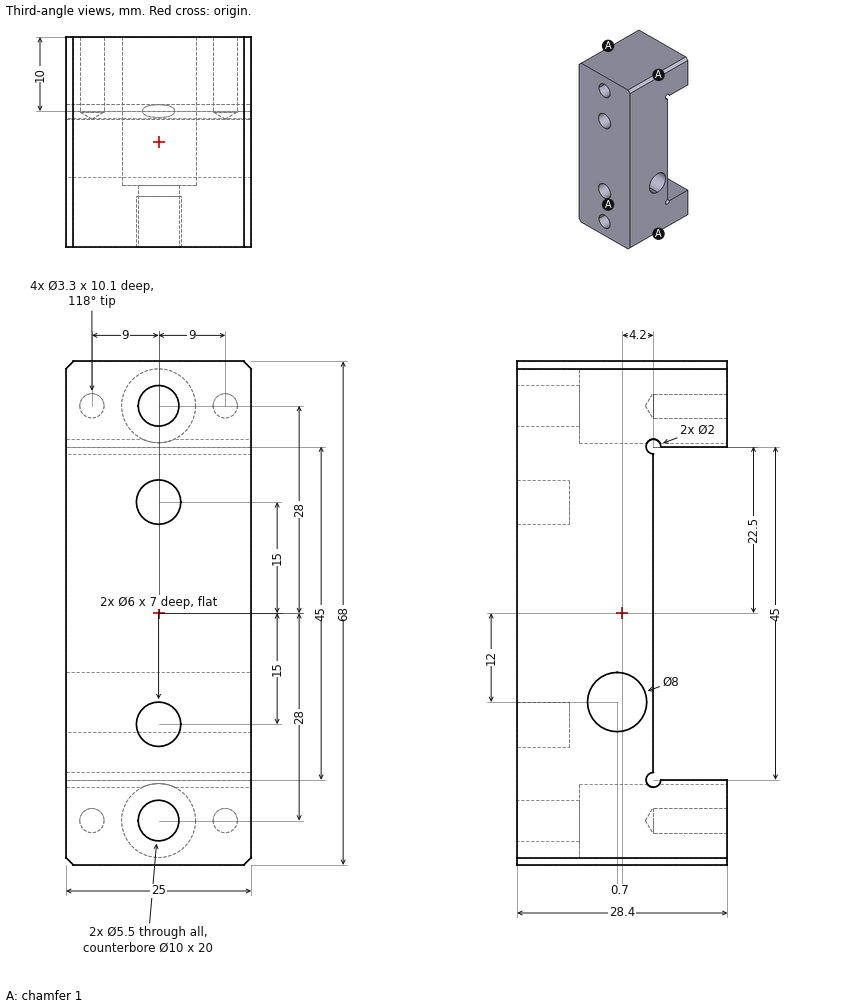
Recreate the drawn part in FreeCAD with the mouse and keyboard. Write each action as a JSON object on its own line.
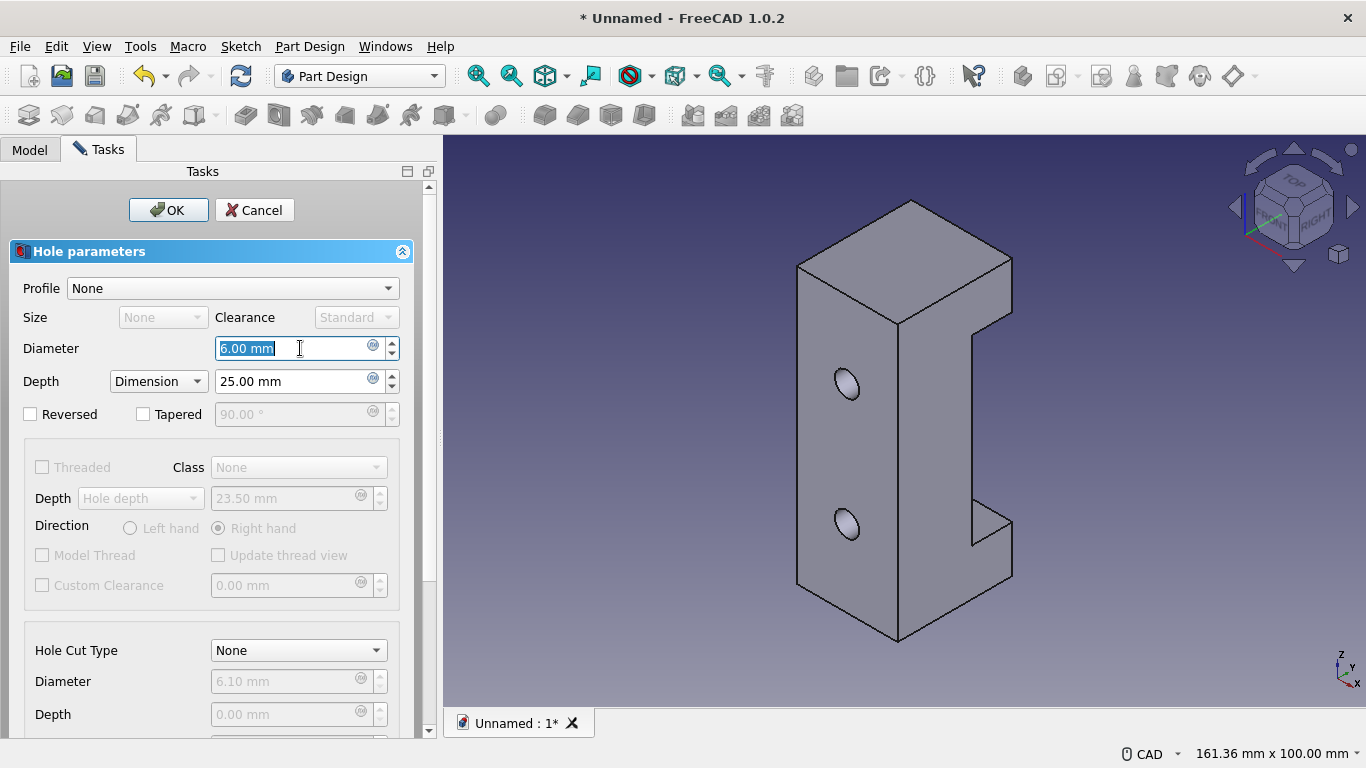
{"action": "type", "text": "6"}
{"action": "key", "text": "Tab"}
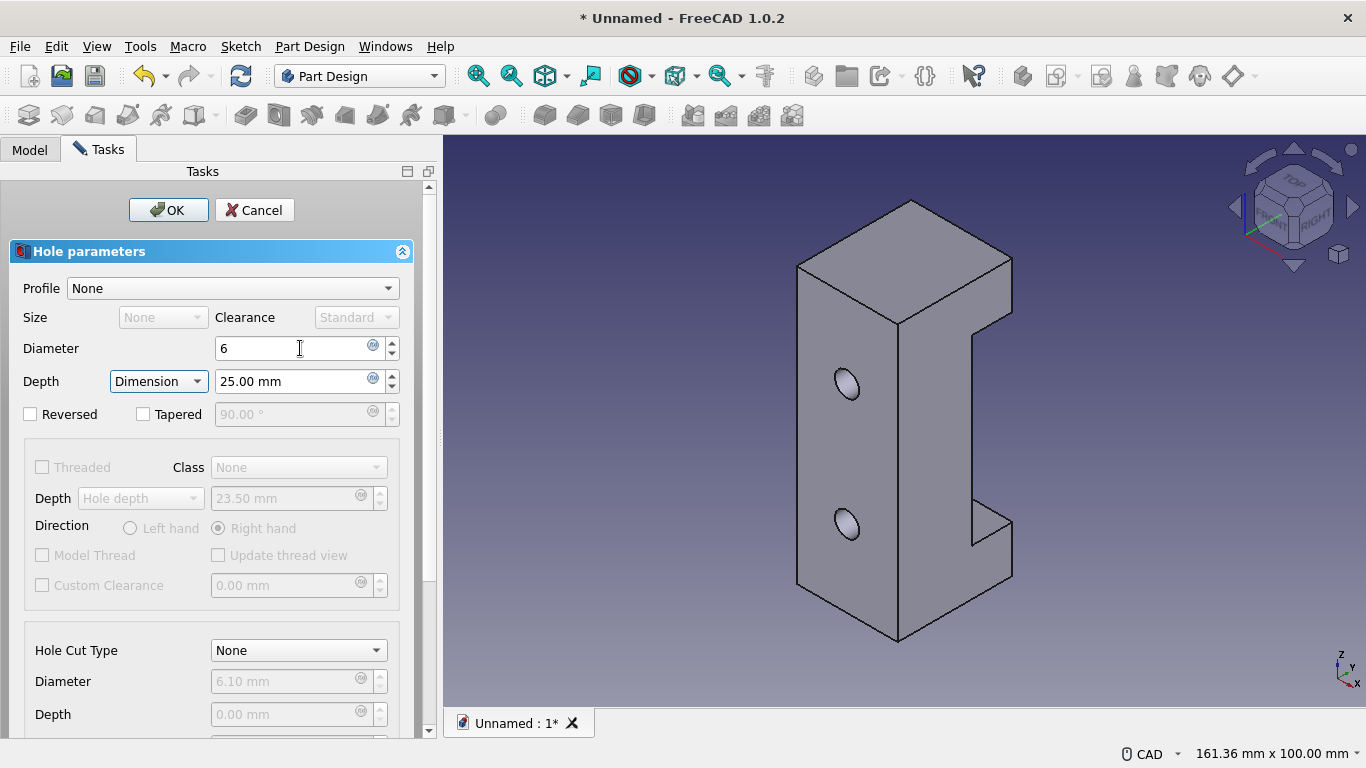
{"action": "triple_click", "coordinate": [300, 382]}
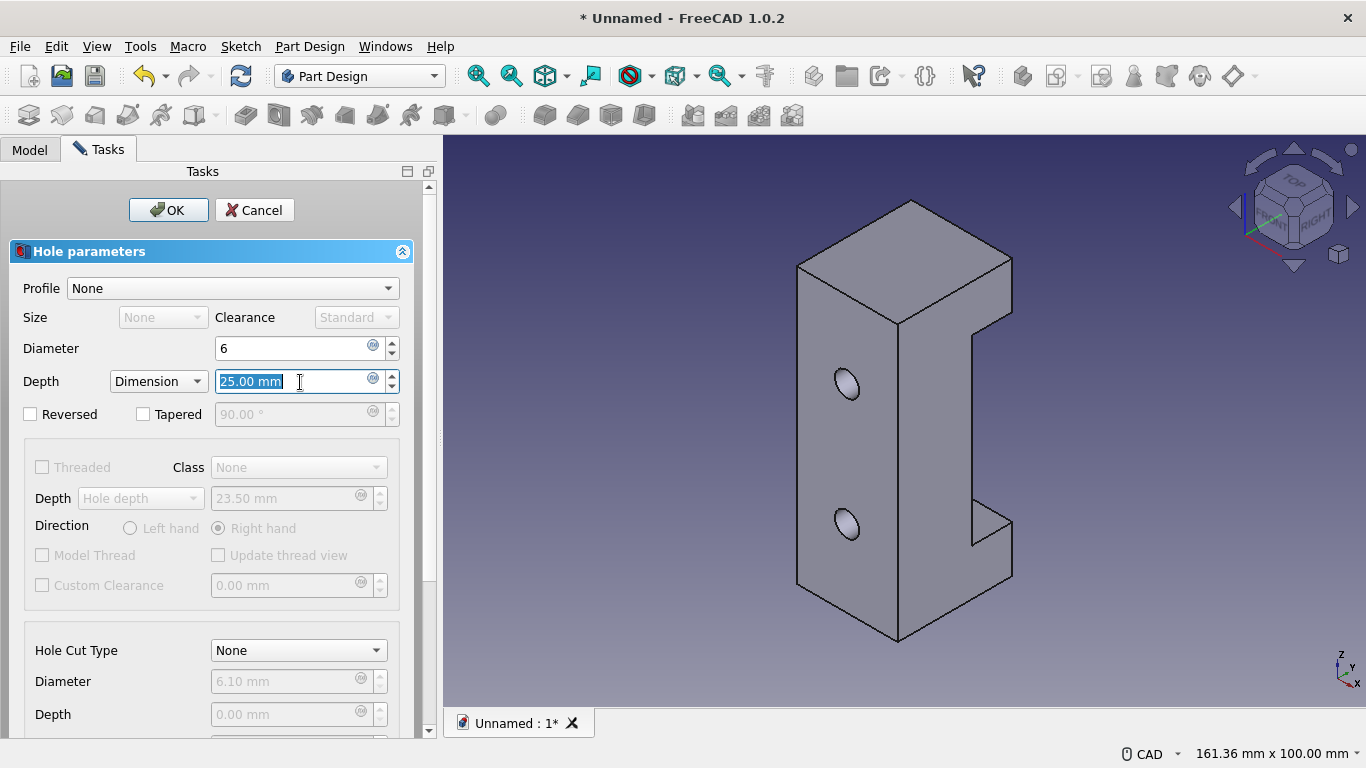
{"action": "type", "text": "7"}
{"action": "key", "text": "Tab"}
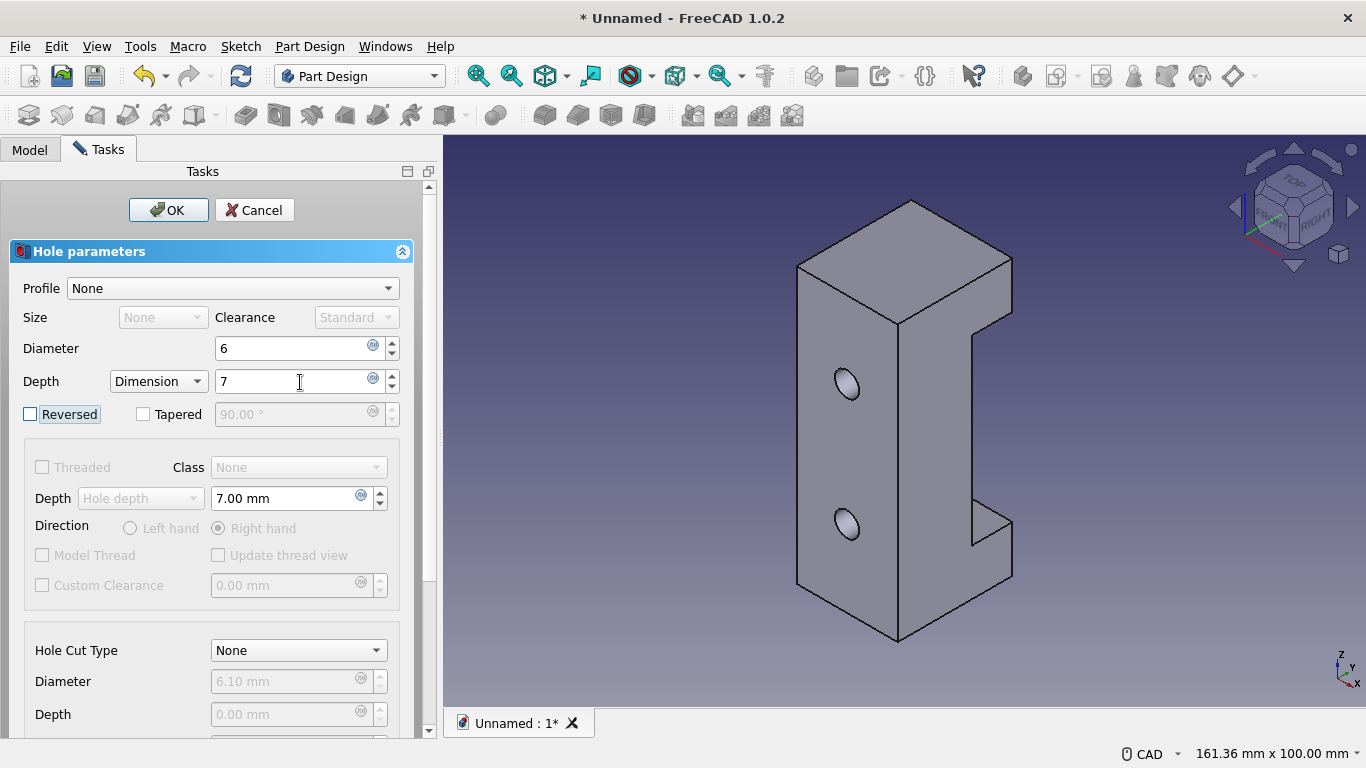
{"action": "scroll", "coordinate": [429, 460], "scroll_direction": "down", "scroll_amount": 3}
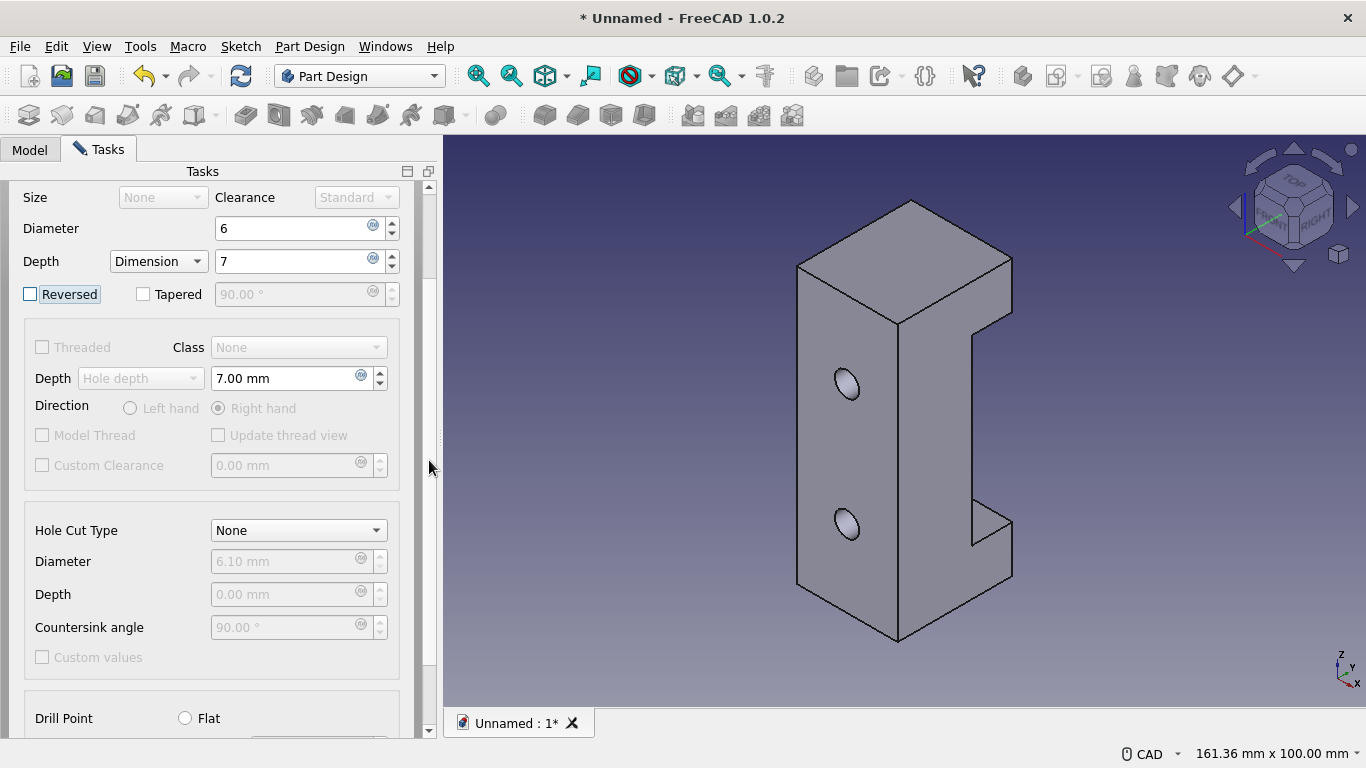
{"action": "left_click", "coordinate": [186, 656]}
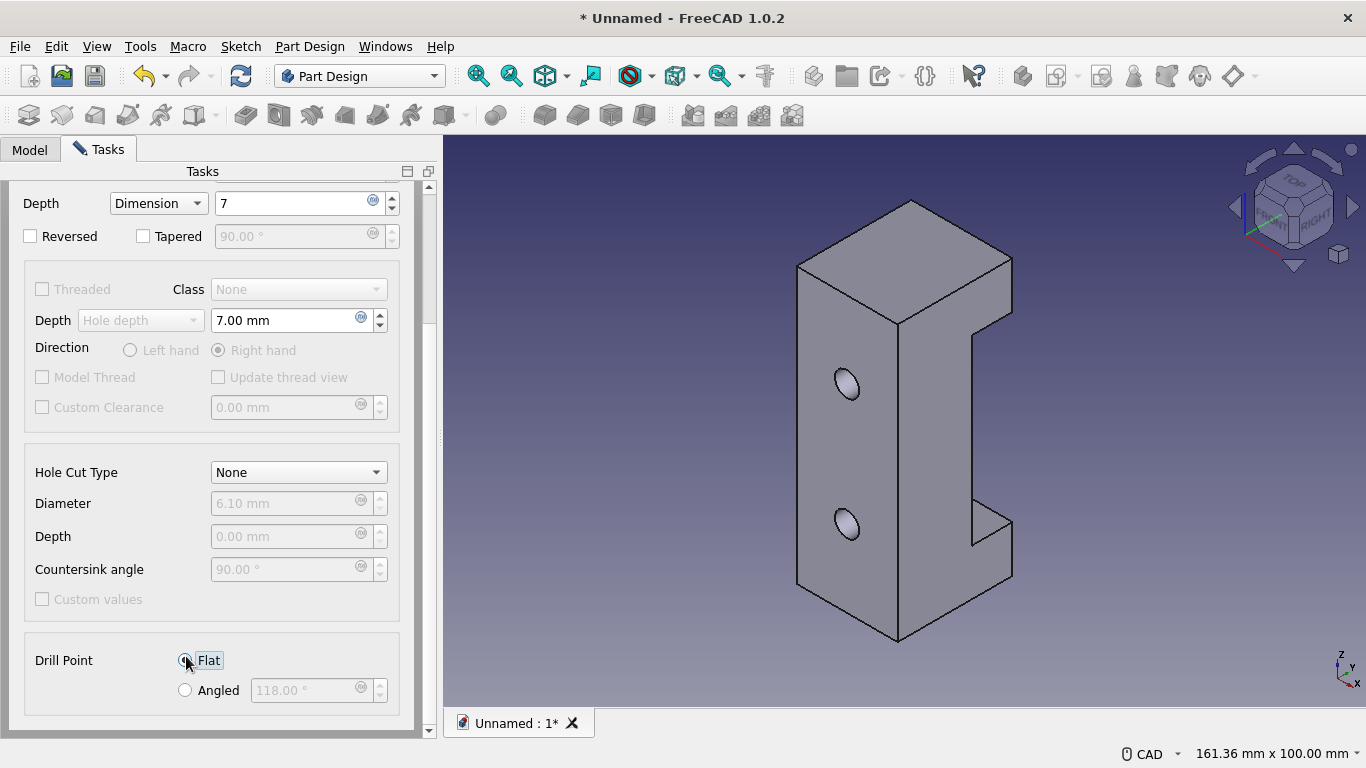
{"action": "scroll", "coordinate": [429, 460], "scroll_direction": "up", "scroll_amount": 4}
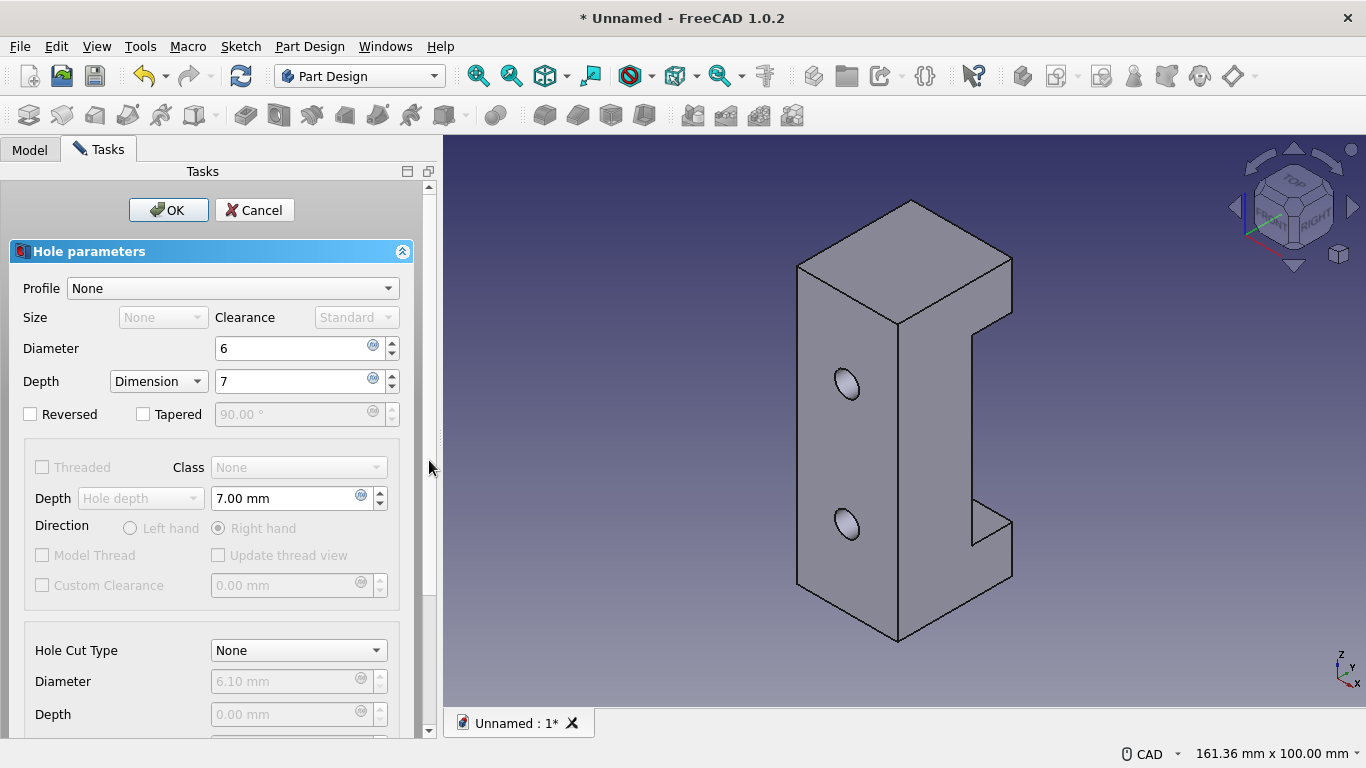
{"action": "left_click", "coordinate": [169, 210]}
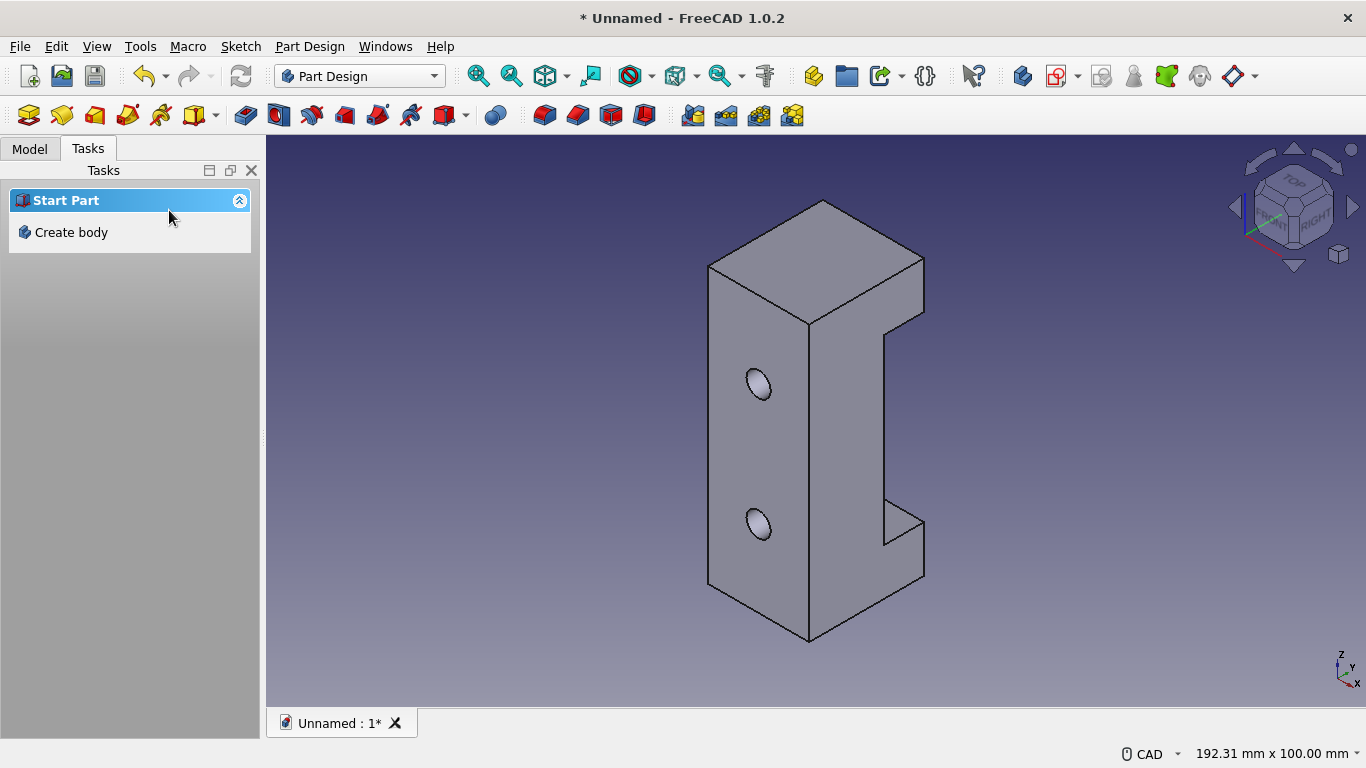
{"action": "key", "text": "4"}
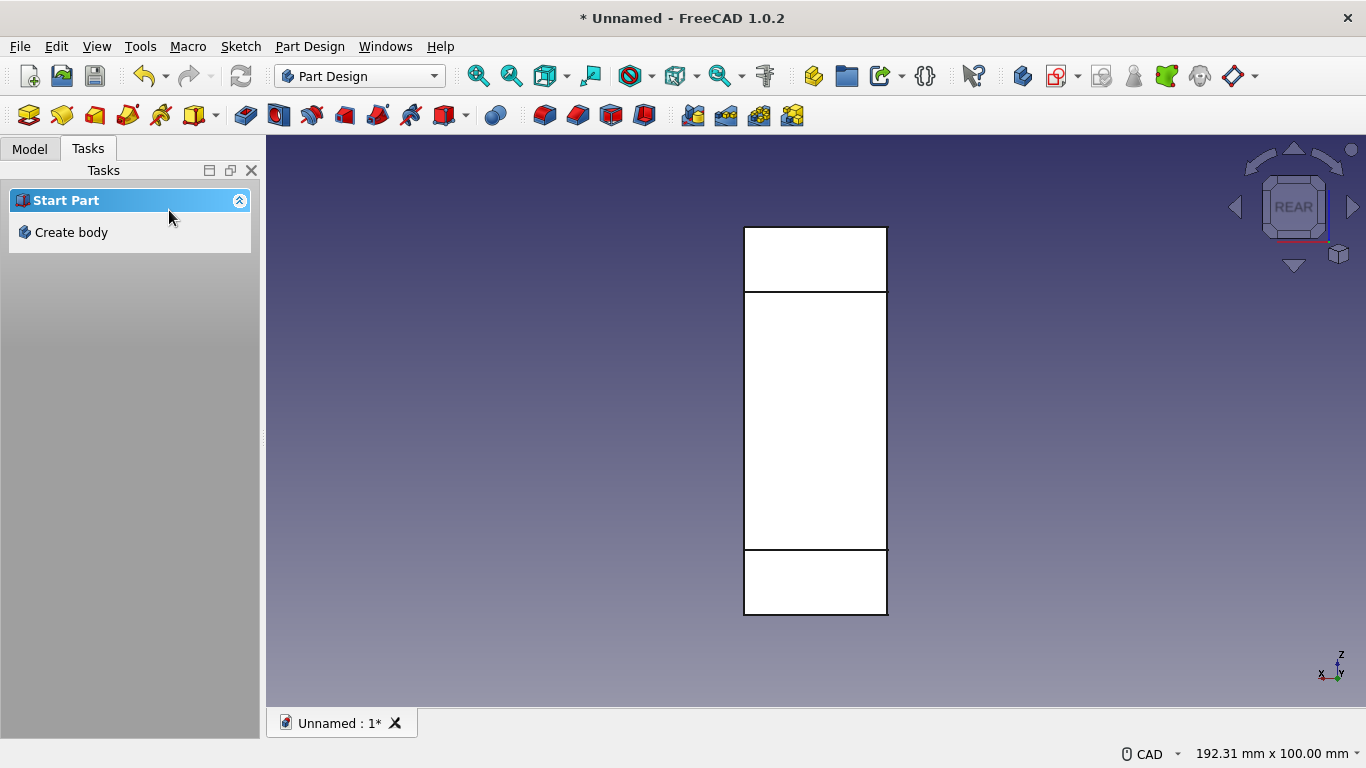
{"action": "left_click", "coordinate": [796, 582]}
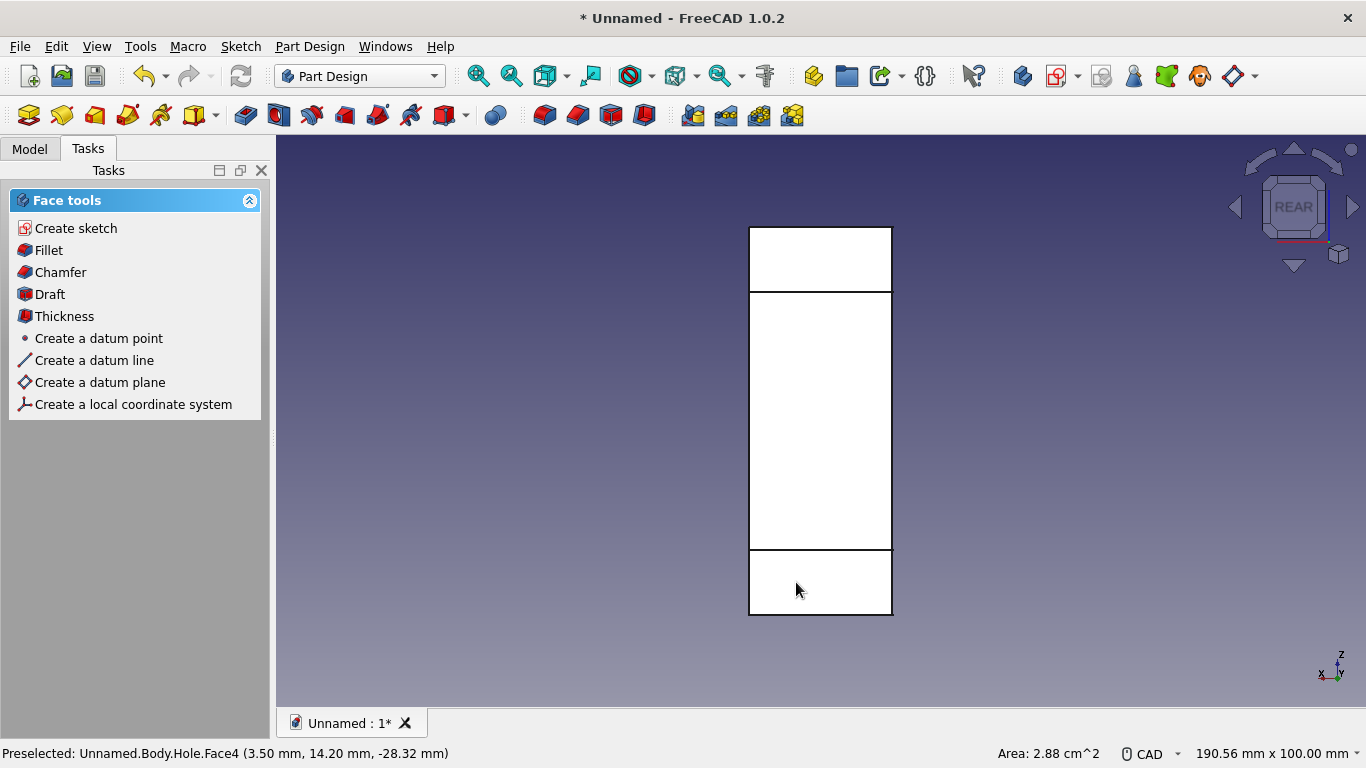
{"action": "left_click", "coordinate": [1056, 76]}